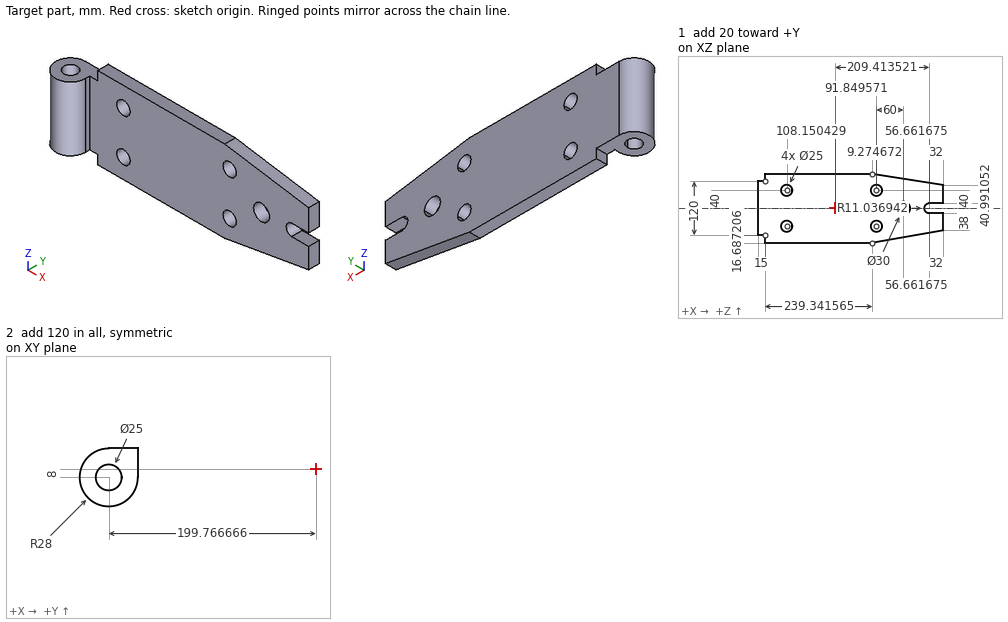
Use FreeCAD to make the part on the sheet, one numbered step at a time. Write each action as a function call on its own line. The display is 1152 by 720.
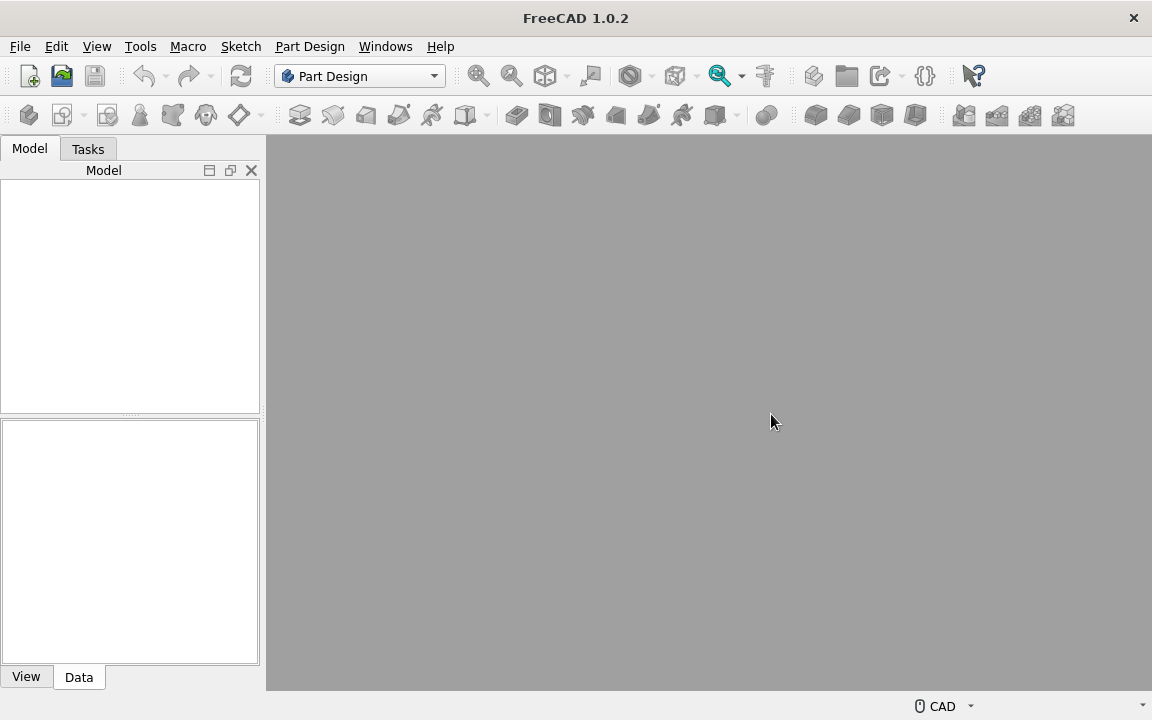
click(29, 76)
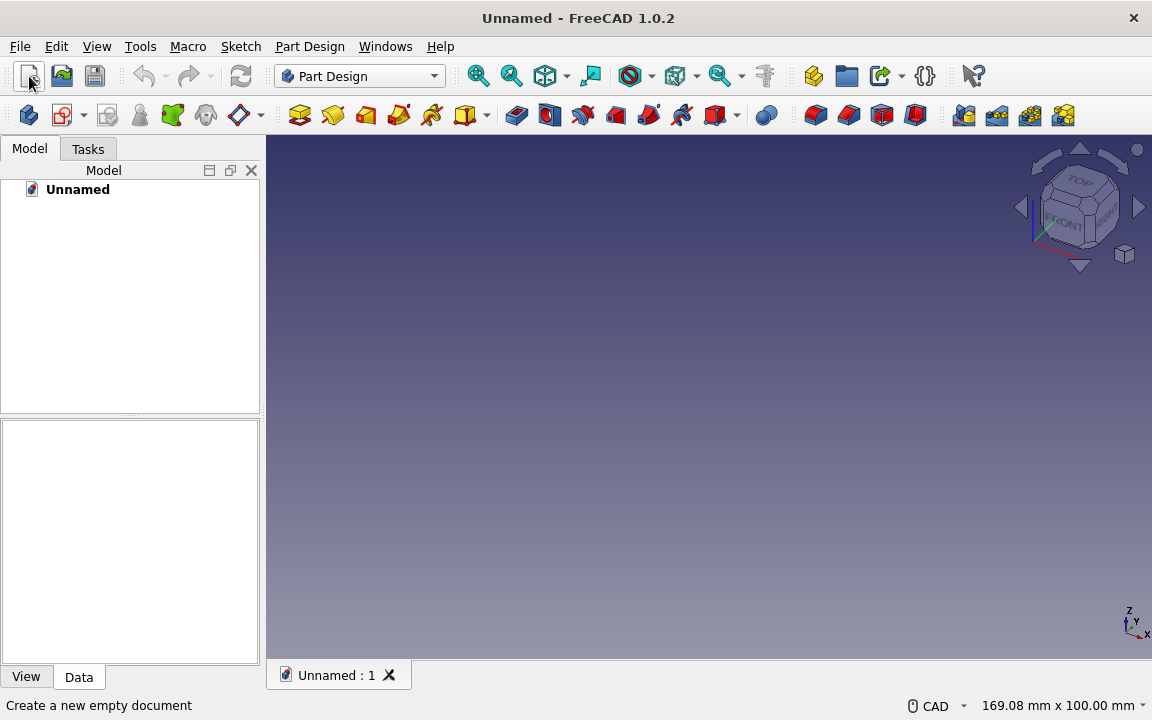
click(62, 116)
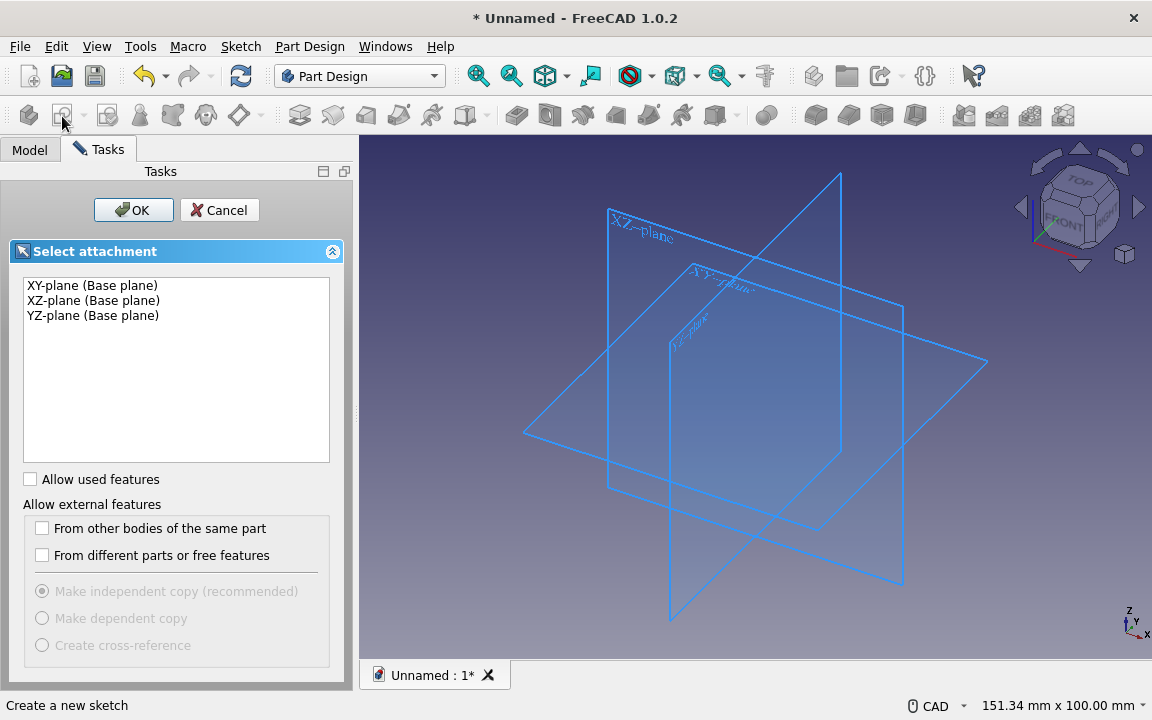
click(84, 300)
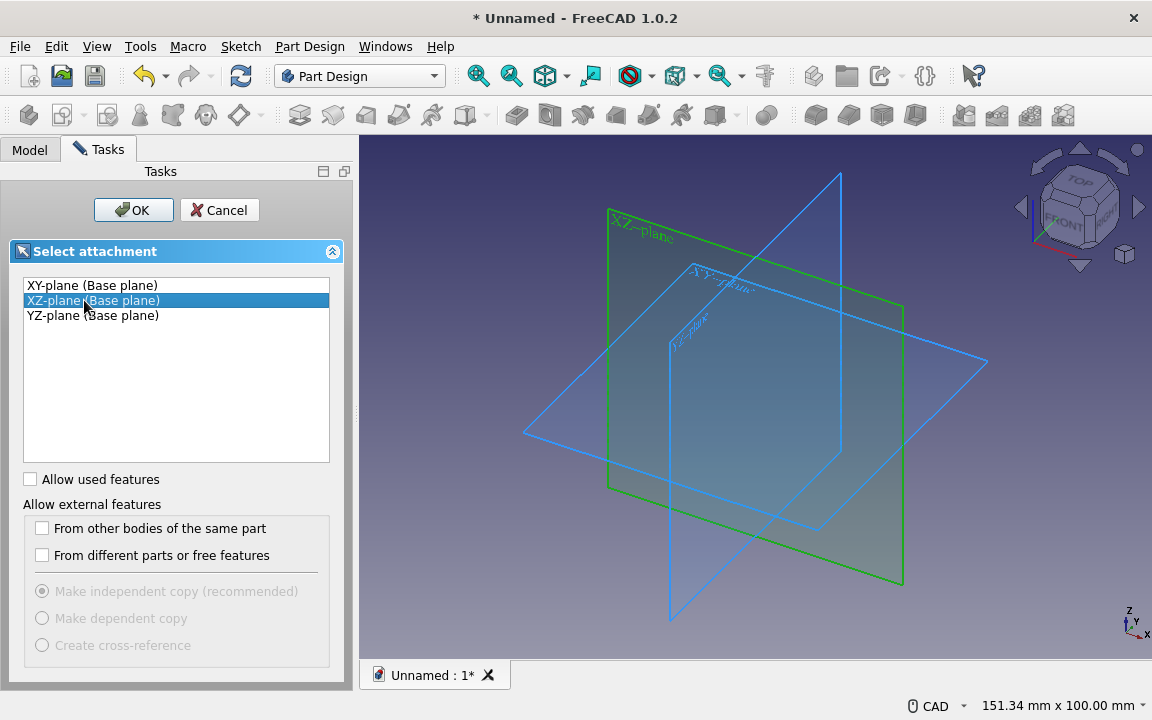
click(134, 210)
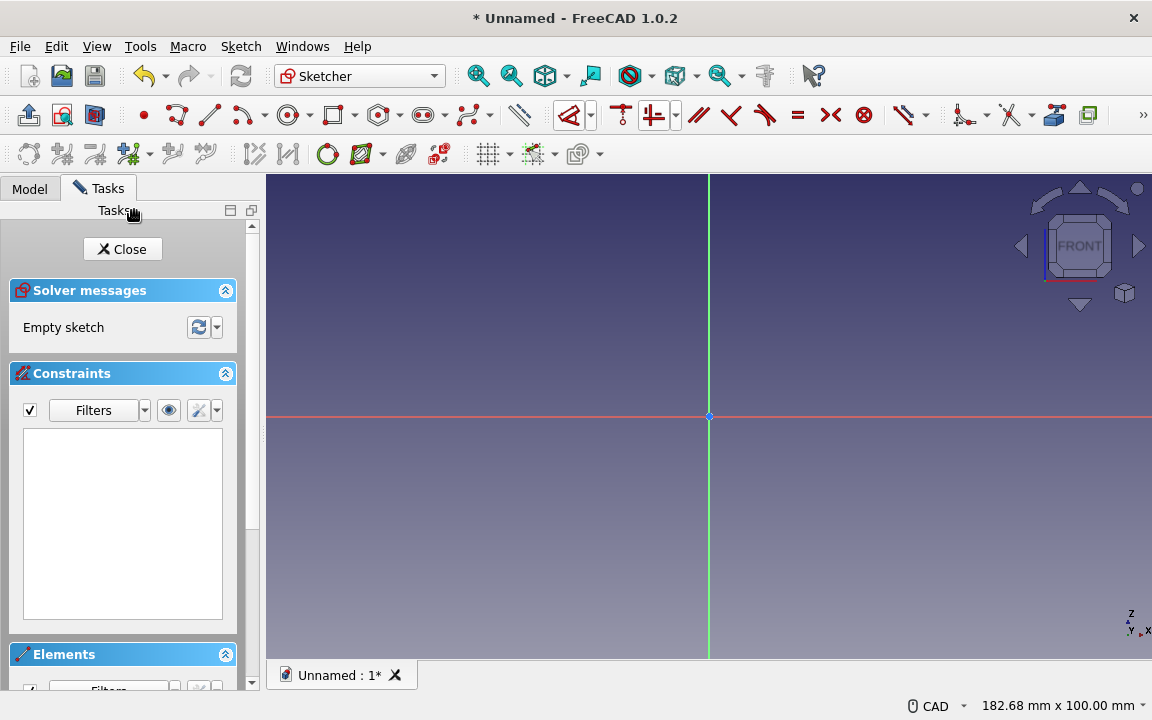
scroll(564, 417, down, 7)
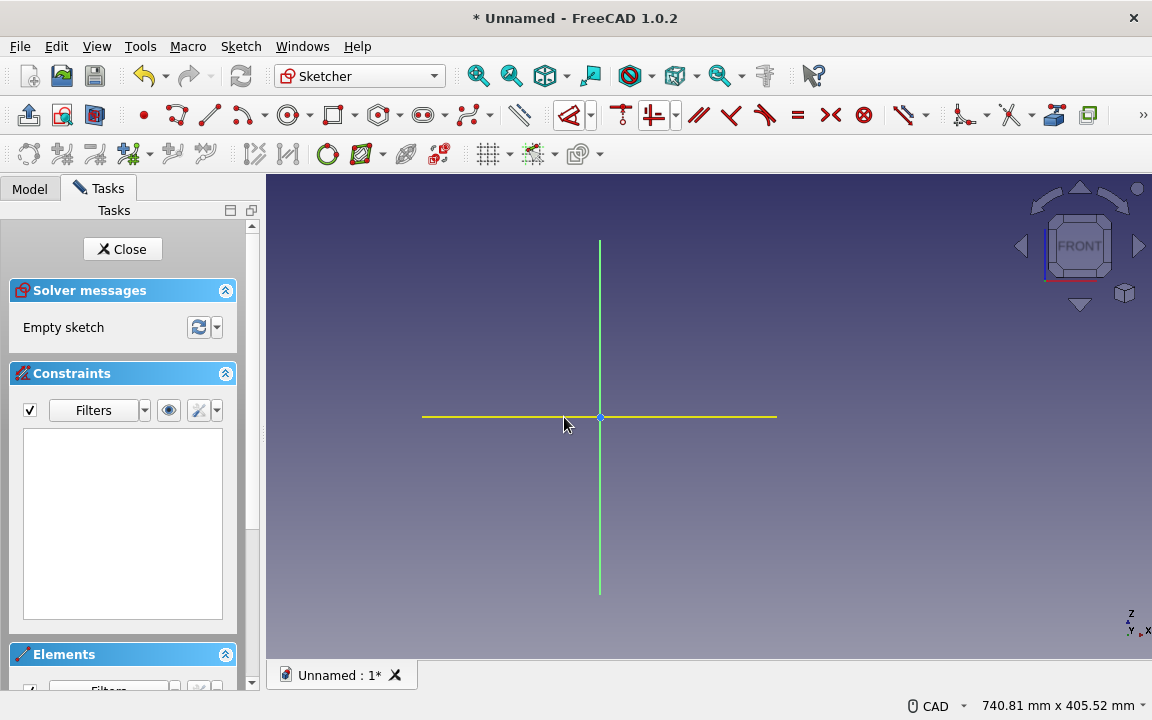
click(177, 116)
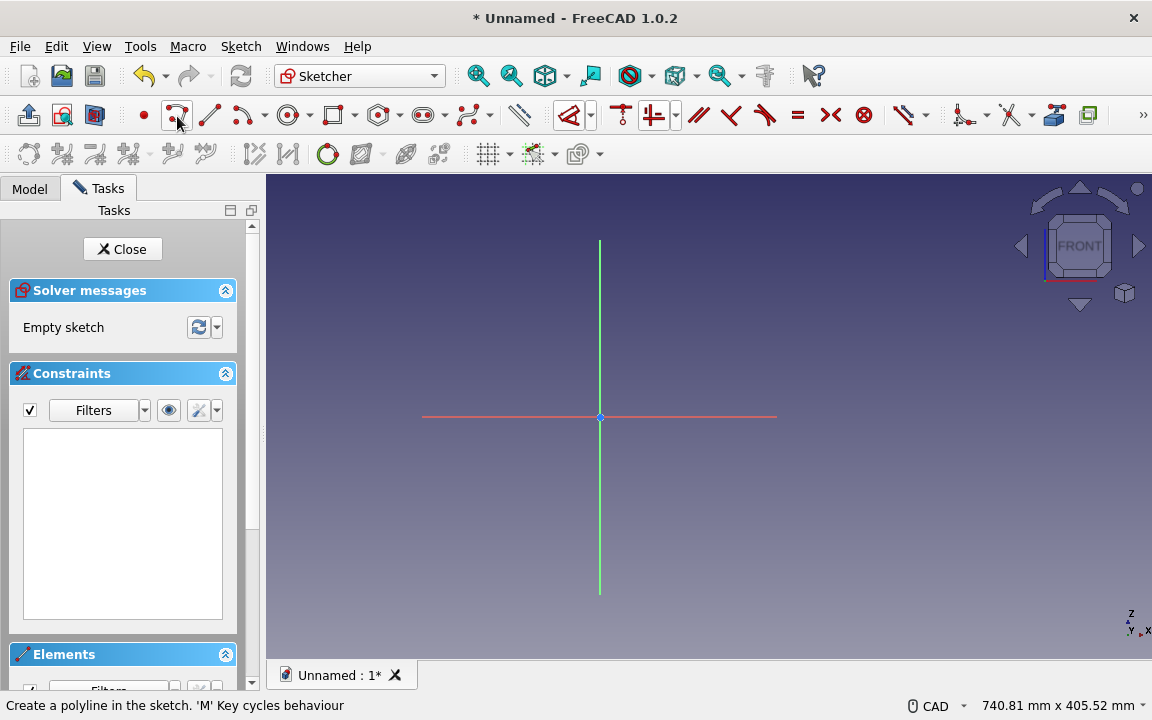
click(849, 430)
click(888, 430)
click(888, 476)
click(699, 509)
click(413, 509)
click(413, 489)
click(395, 489)
click(395, 345)
click(413, 345)
click(413, 326)
click(699, 326)
click(888, 355)
click(888, 404)
click(849, 404)
right_click(849, 404)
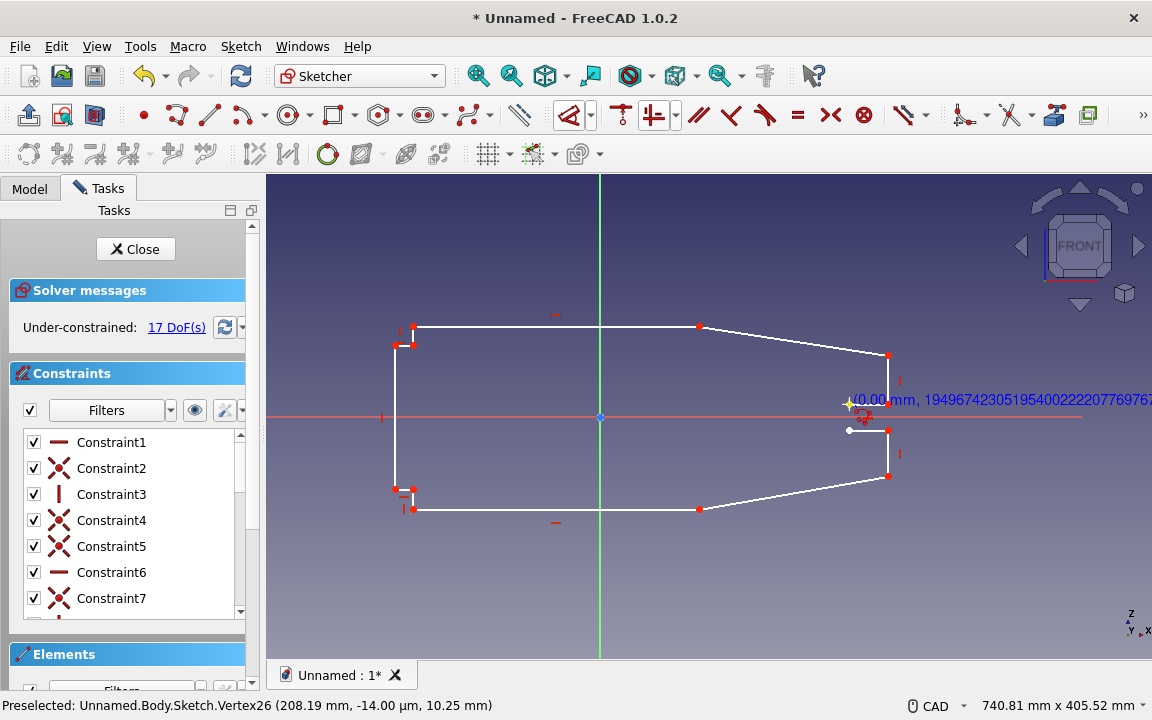
click(264, 116)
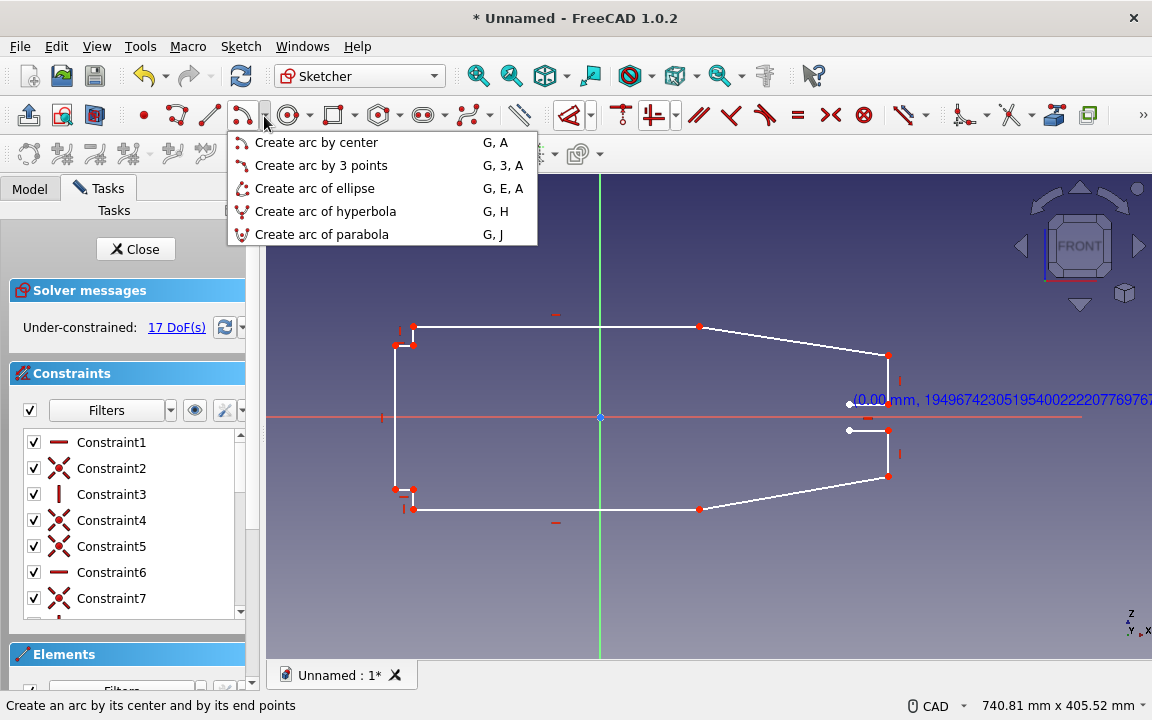
click(382, 166)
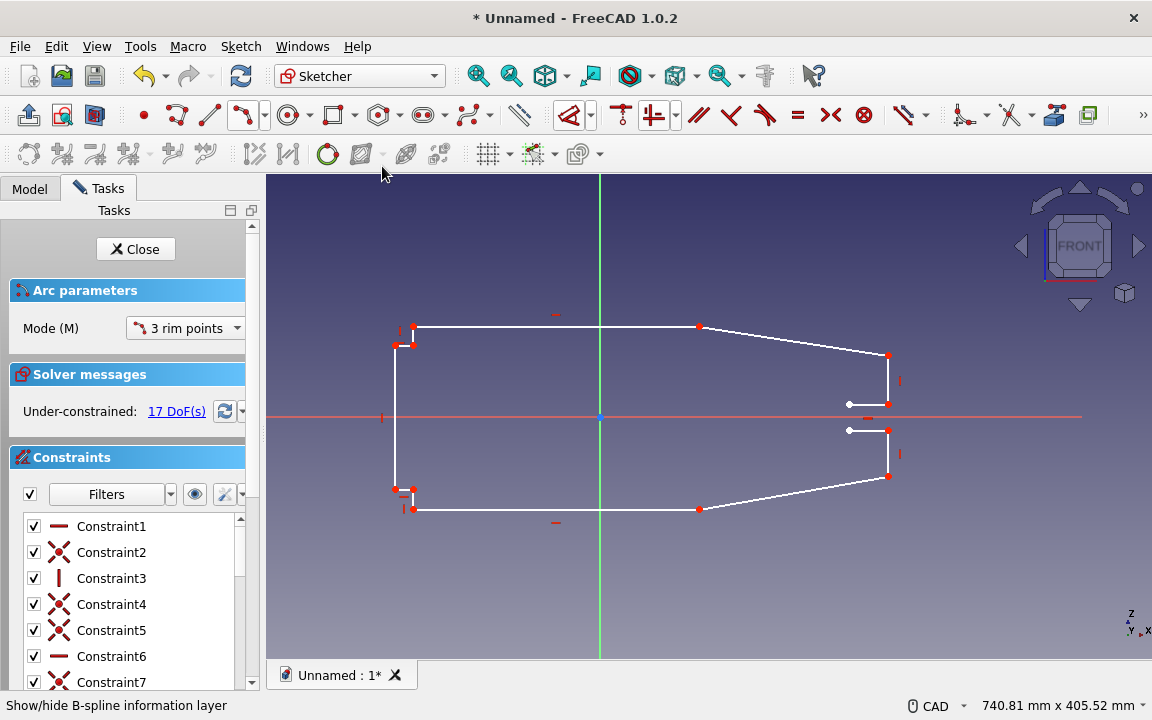
click(849, 405)
click(849, 431)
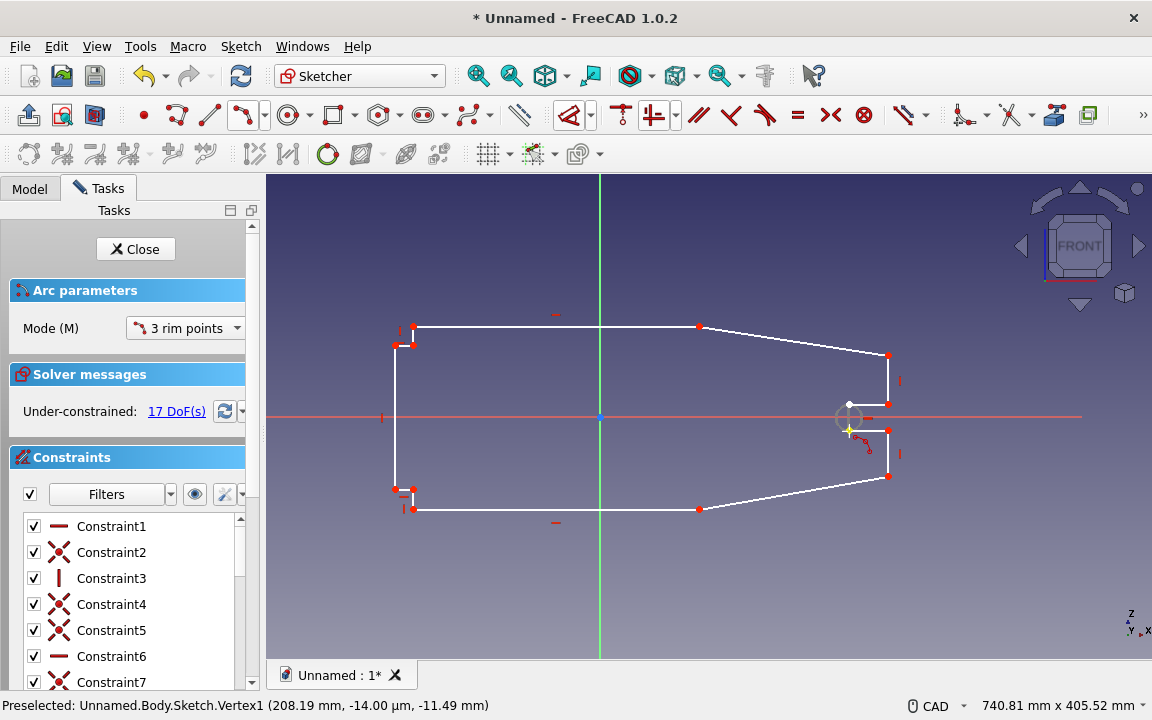
scroll(840, 410, up, 4)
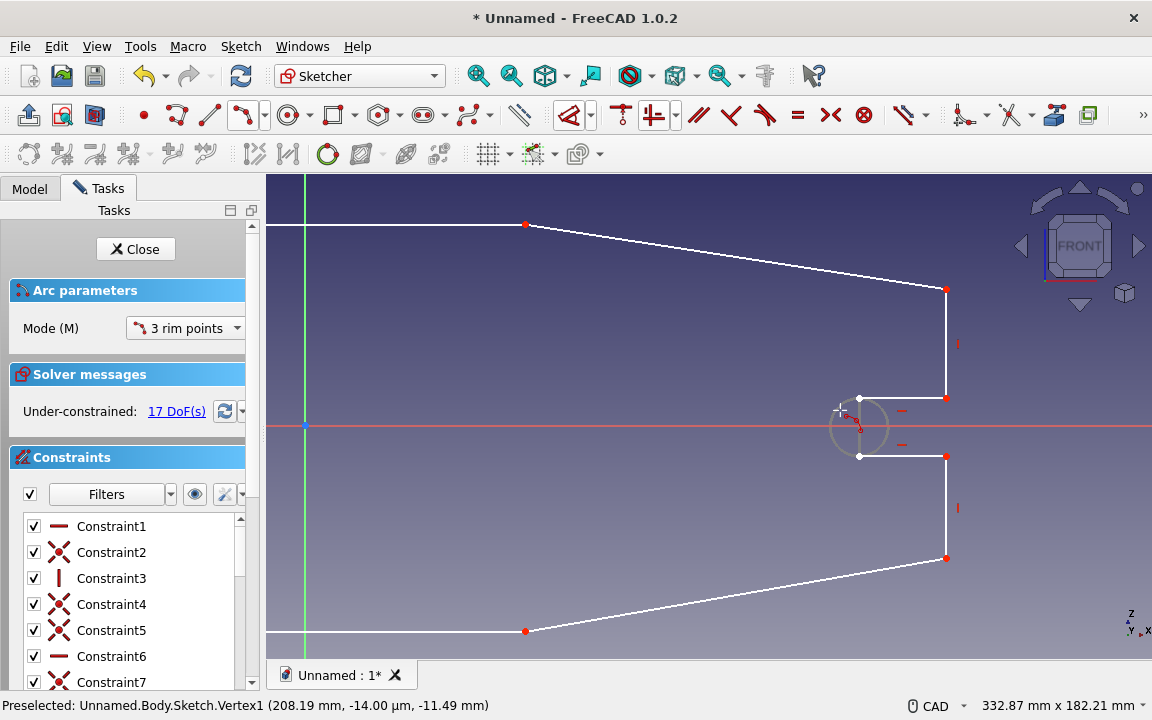
click(838, 409)